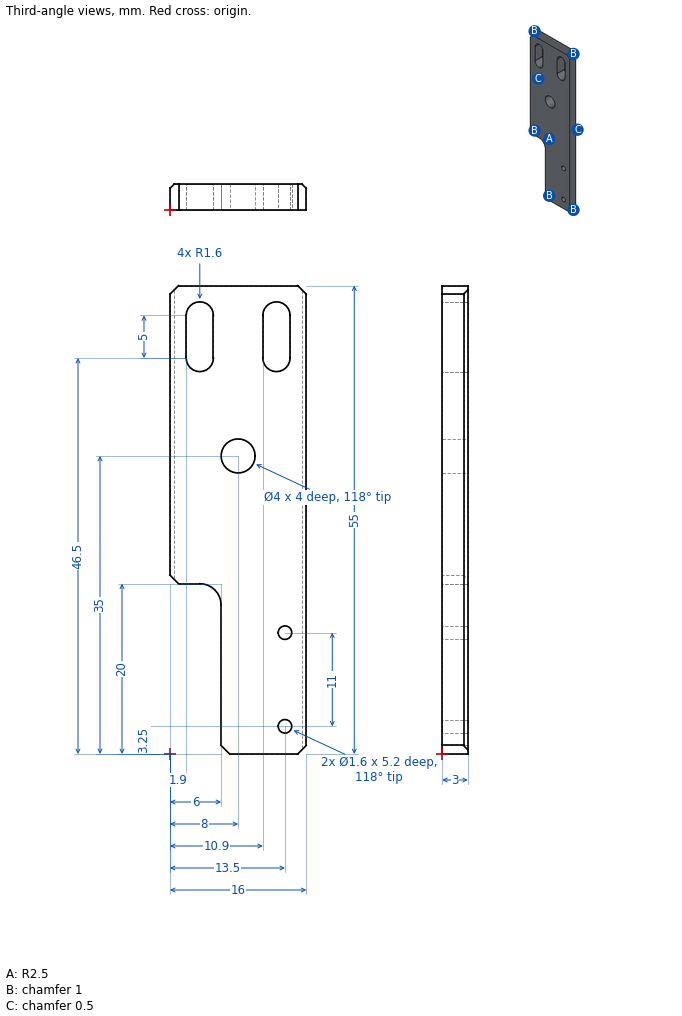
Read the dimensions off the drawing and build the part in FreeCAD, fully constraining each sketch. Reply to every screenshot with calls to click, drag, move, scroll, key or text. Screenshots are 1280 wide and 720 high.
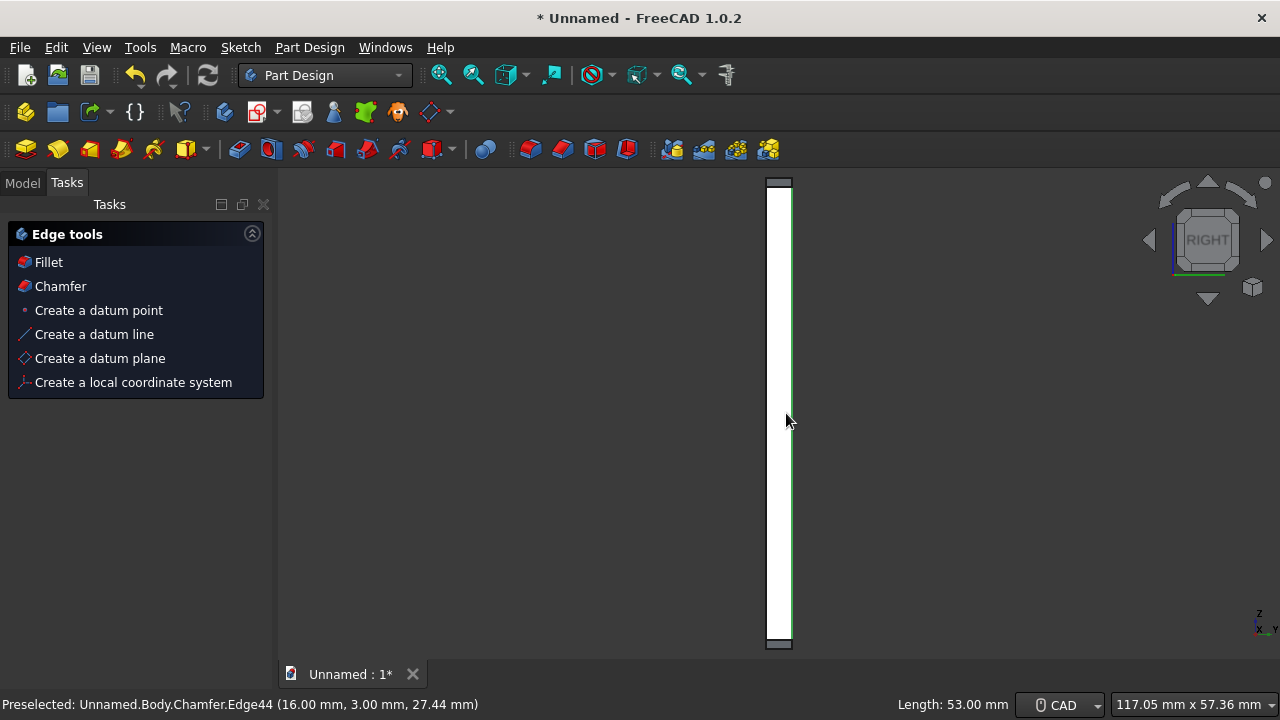
key(5)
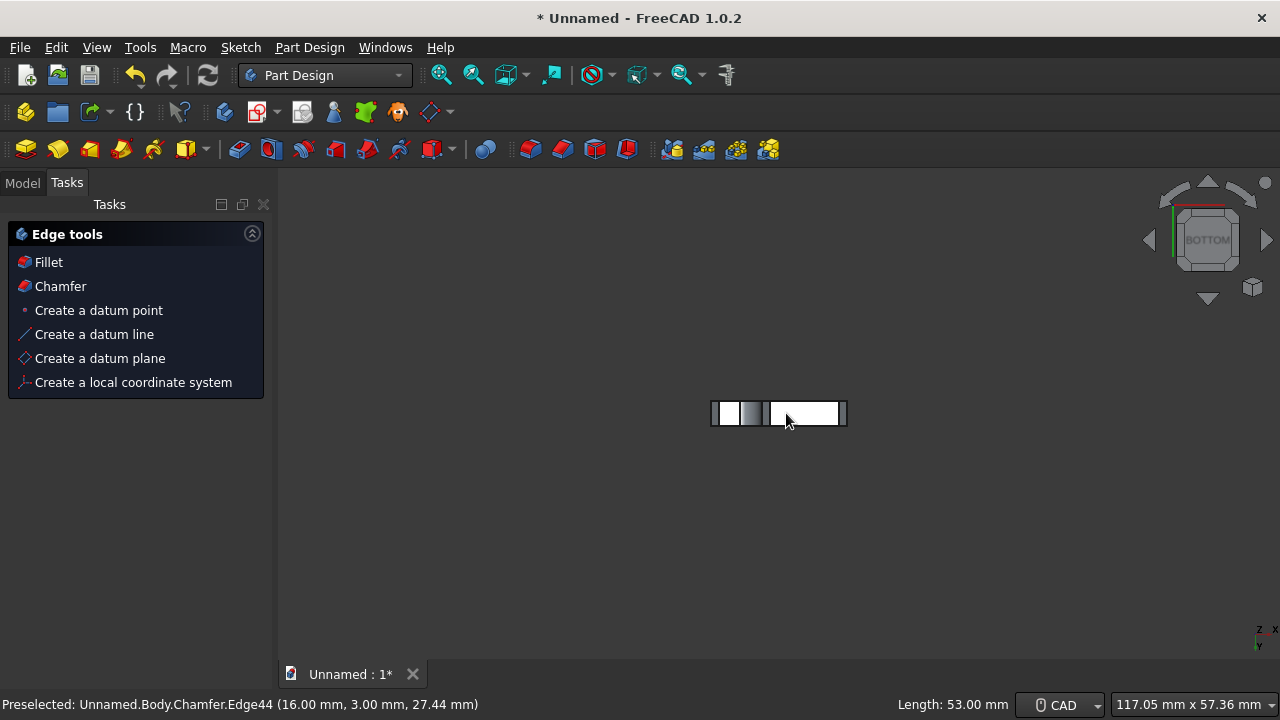
click(442, 76)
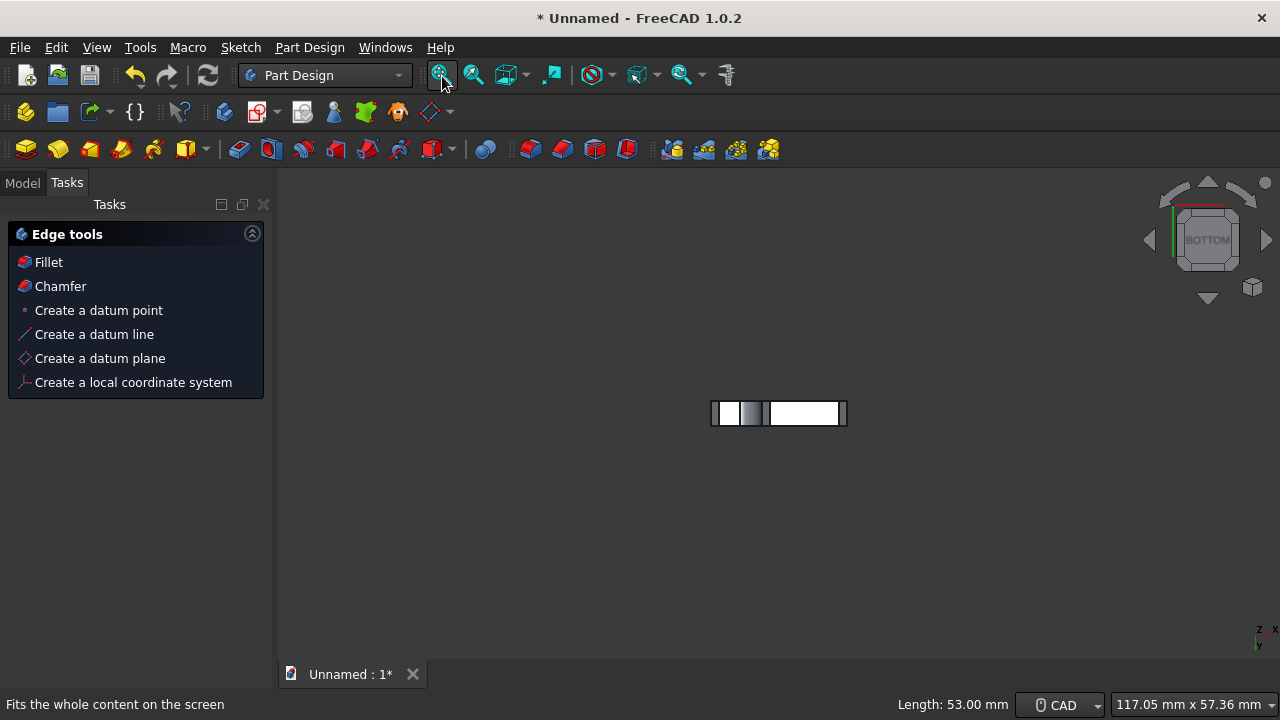
key(4)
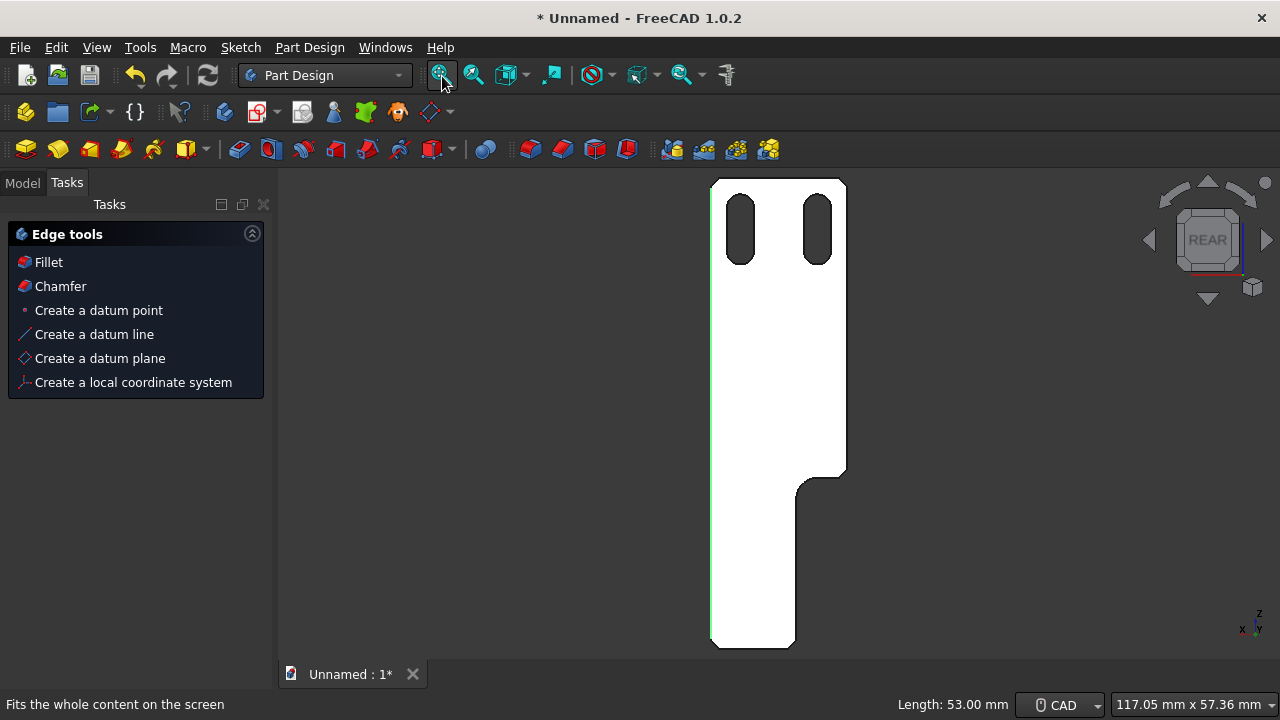
click(847, 327, ctrl)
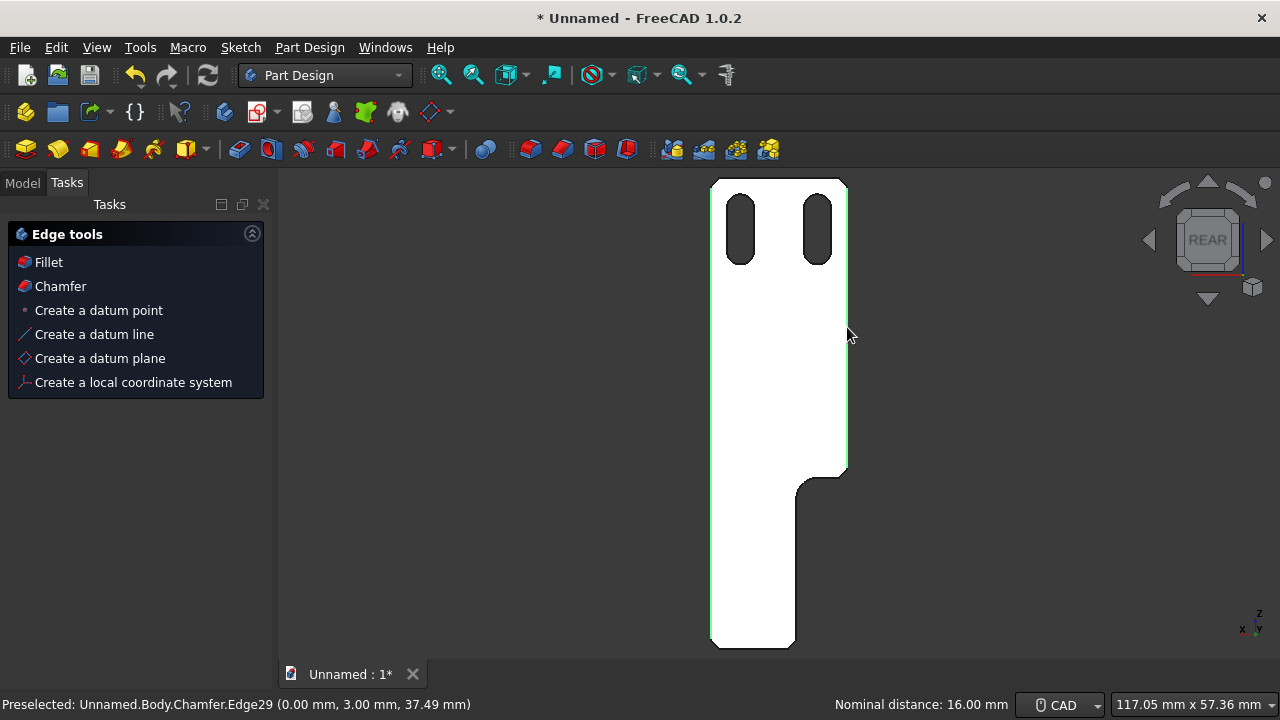
click(564, 150)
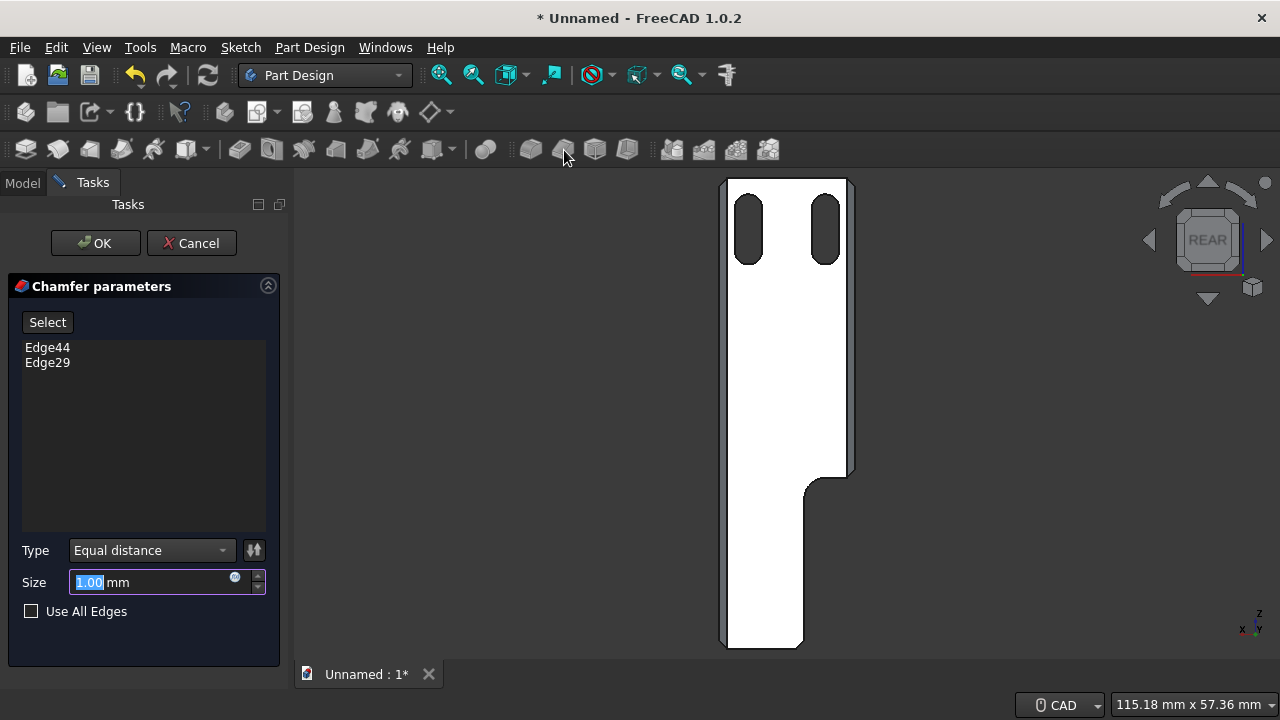
text(0.5)
key(Tab)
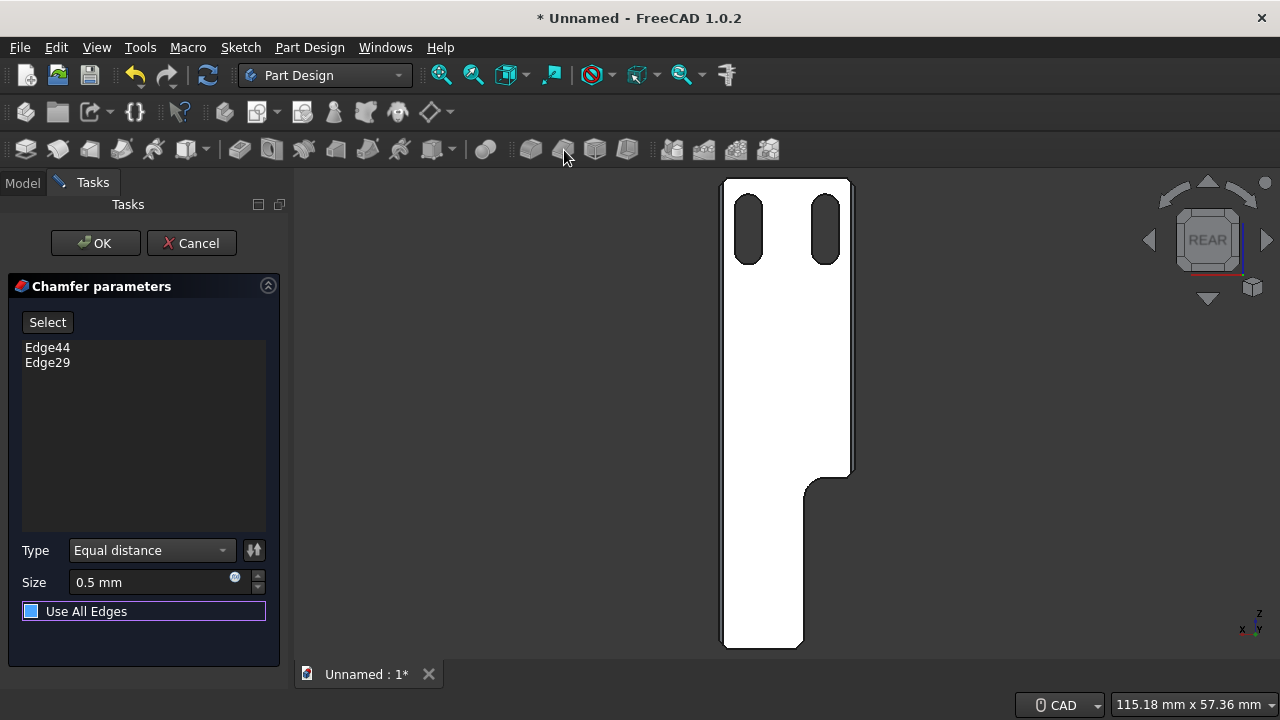
click(96, 243)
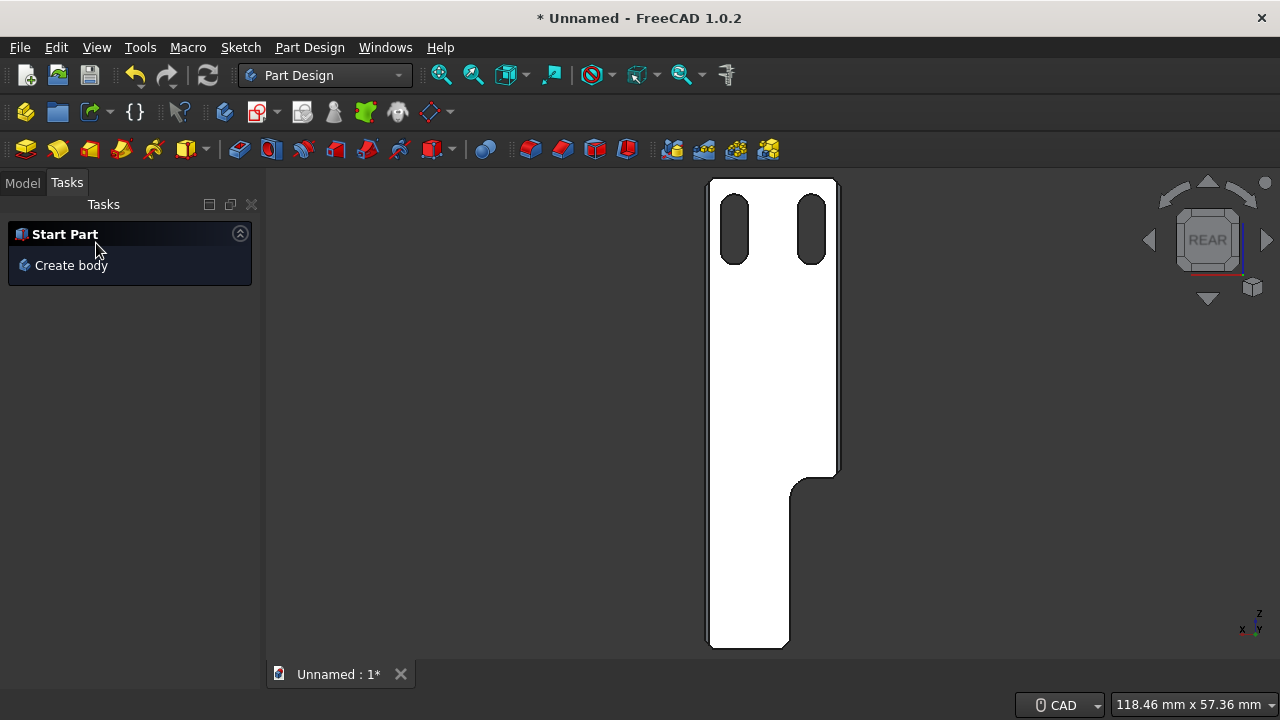
click(773, 345)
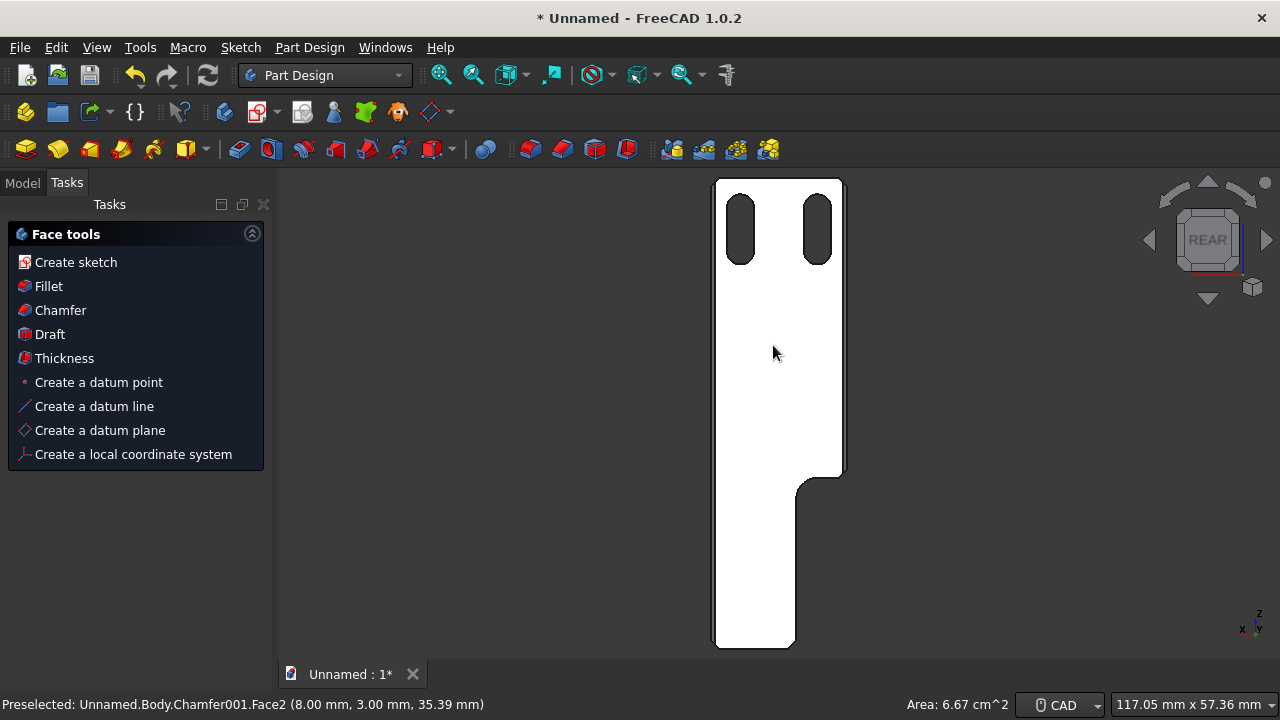
click(258, 112)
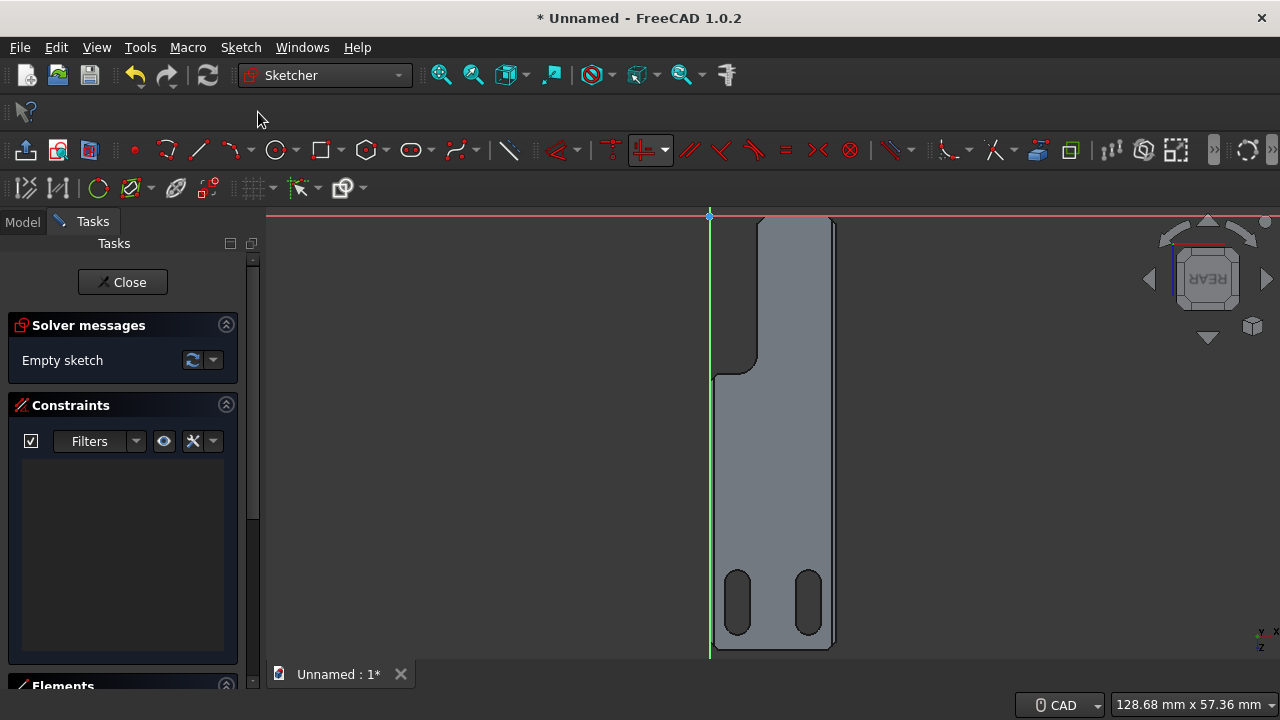
scroll(704, 433, down, 5)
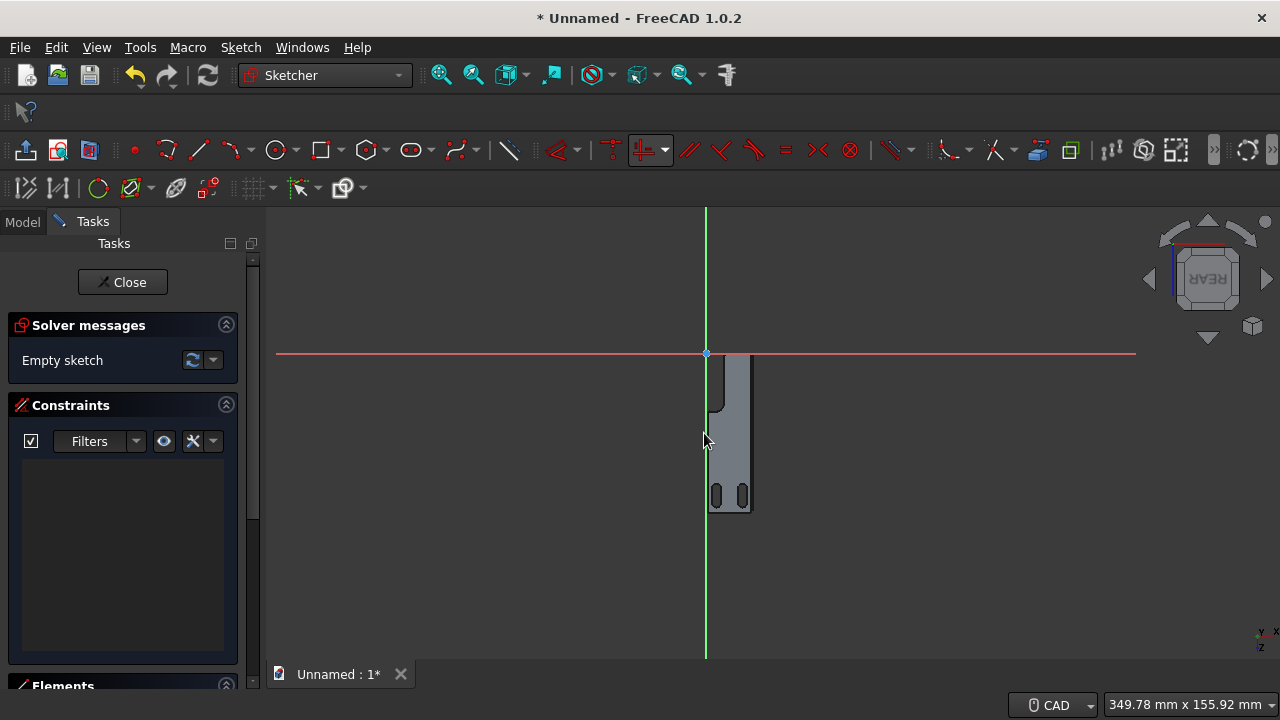
scroll(732, 364, up, 9)